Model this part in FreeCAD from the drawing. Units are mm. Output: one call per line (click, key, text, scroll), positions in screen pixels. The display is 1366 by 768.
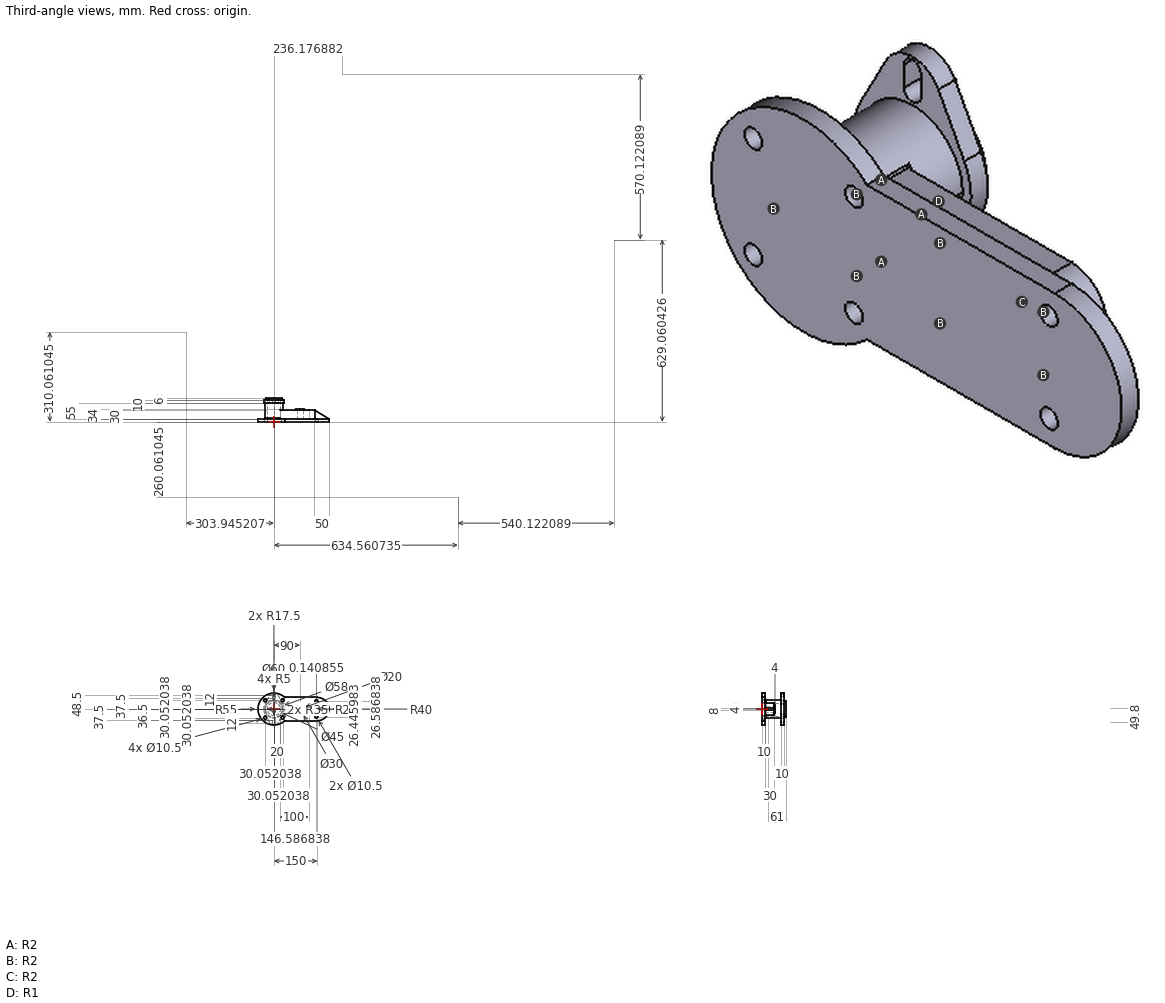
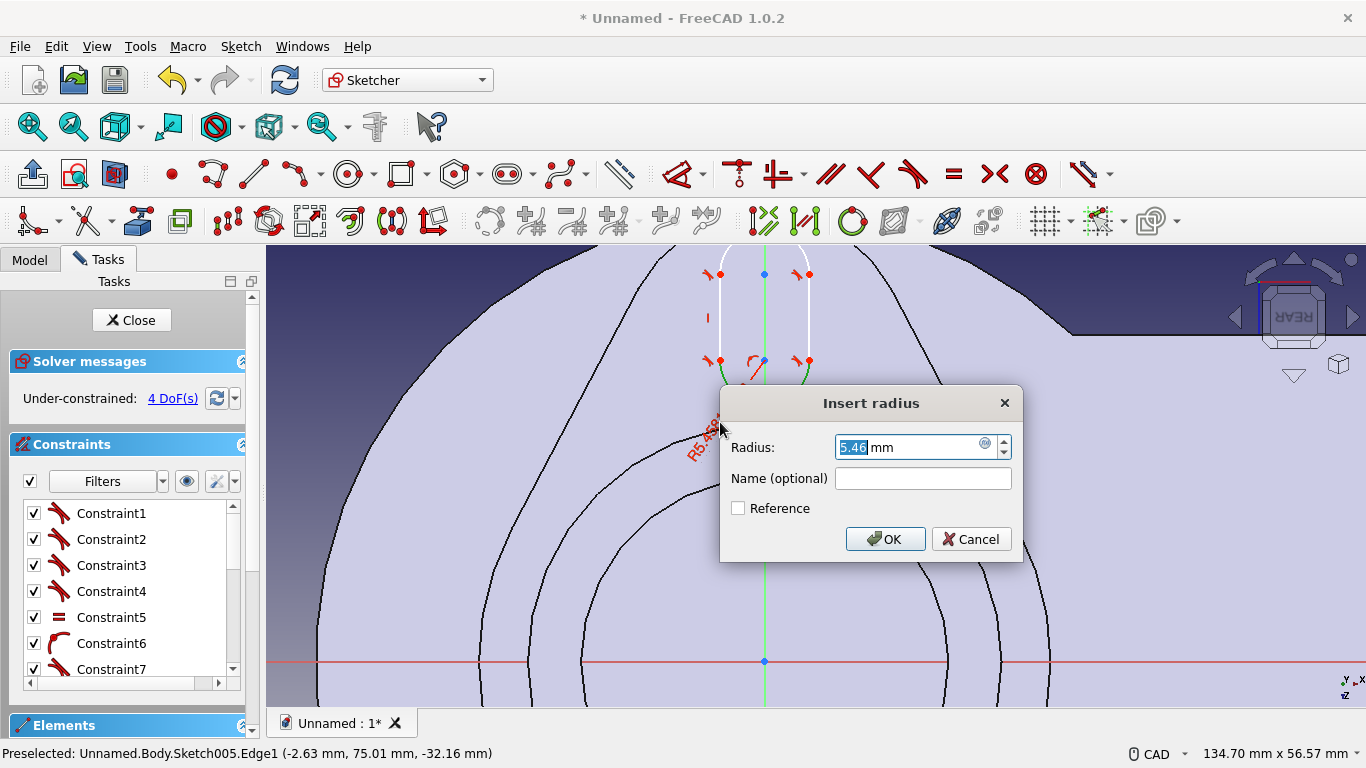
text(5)
key(Return)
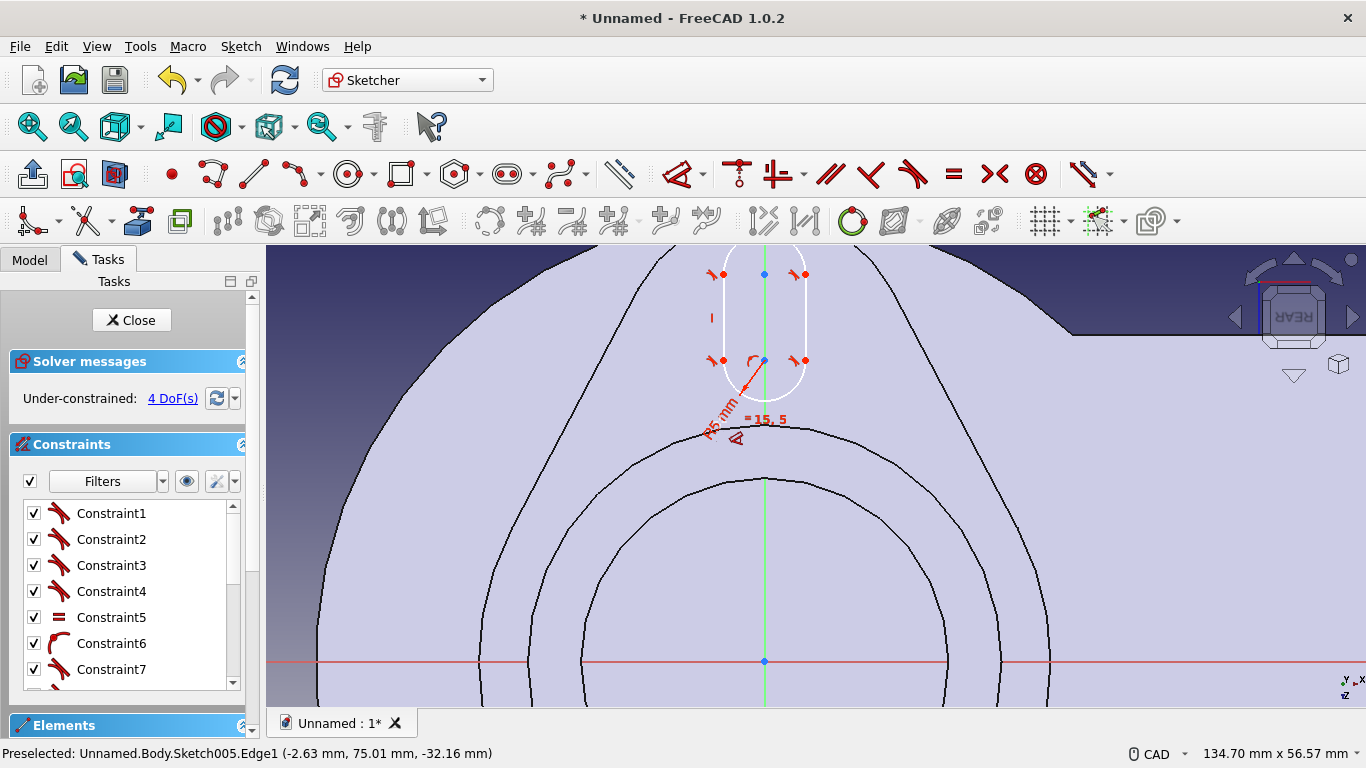
click(724, 334)
click(690, 317)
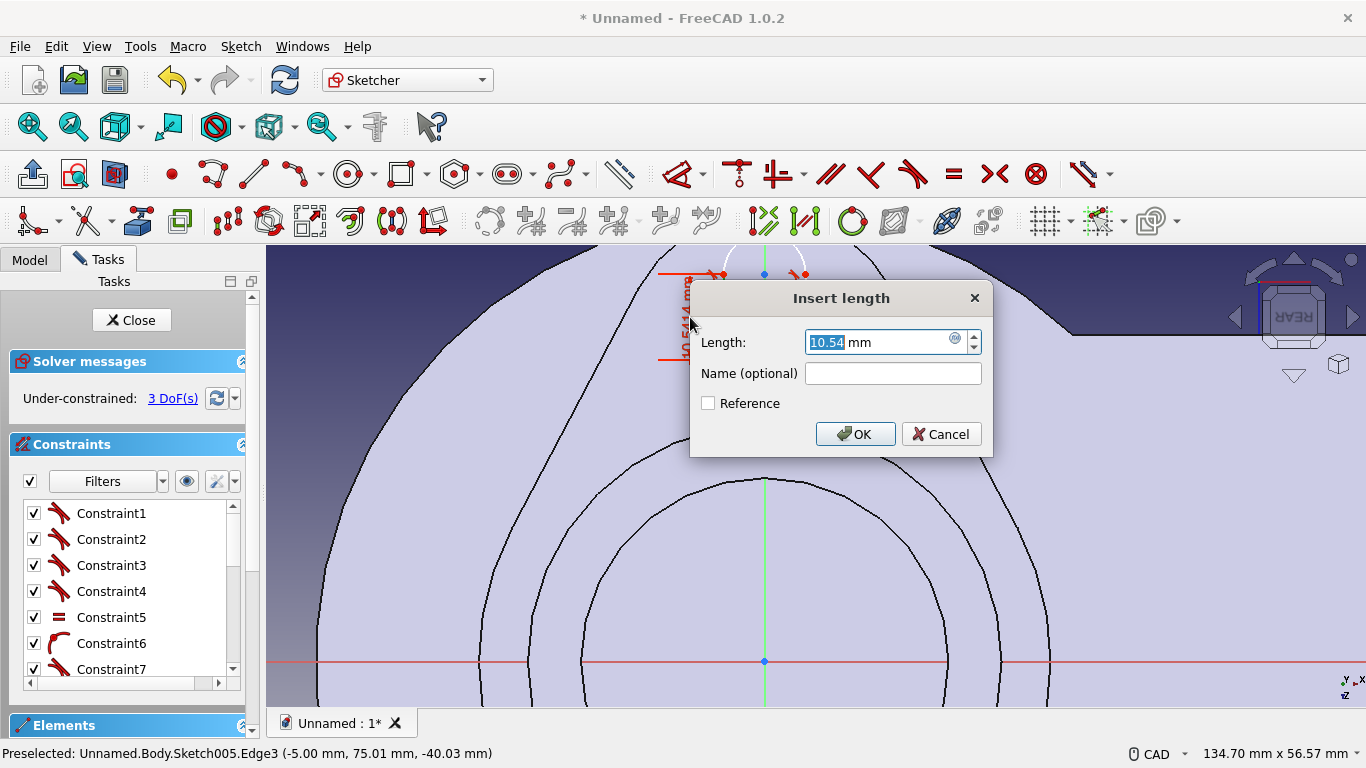
text(12)
key(Return)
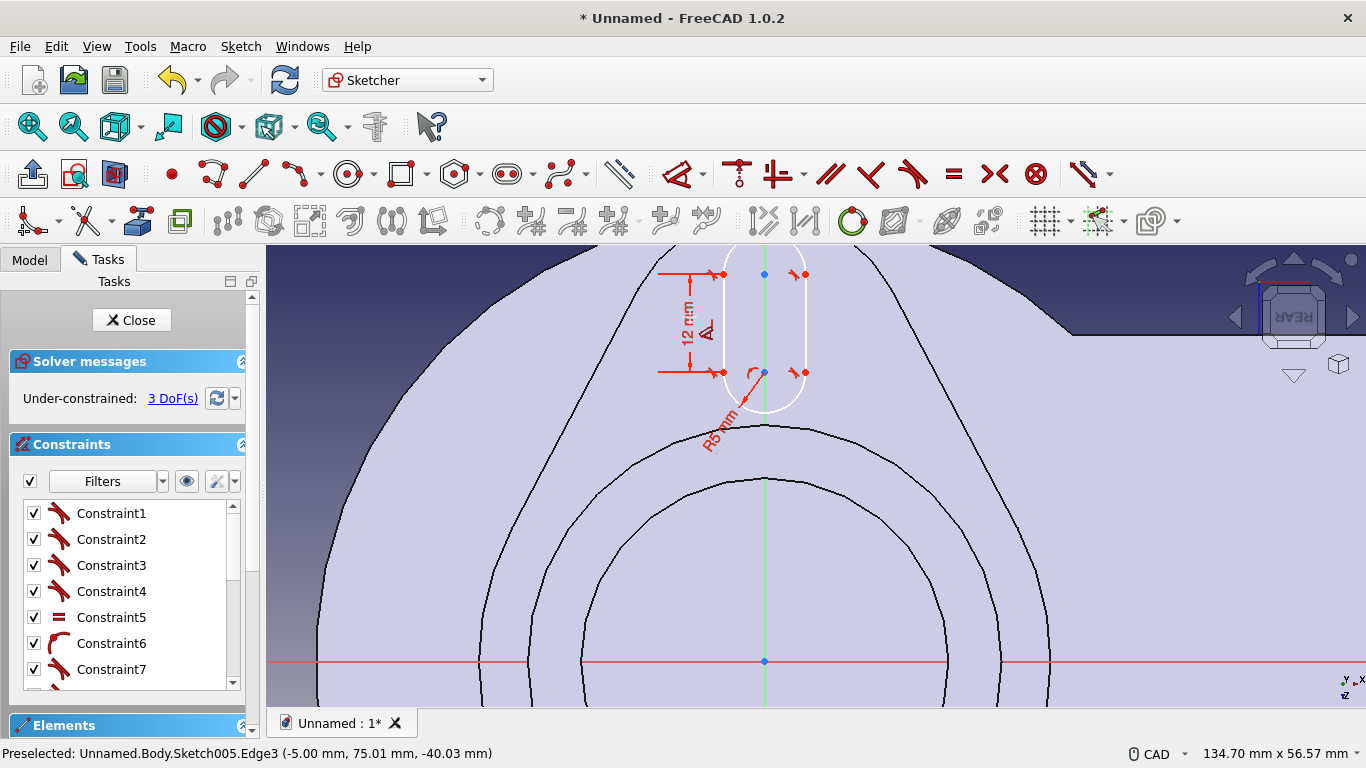
scroll(740, 396, down, 6)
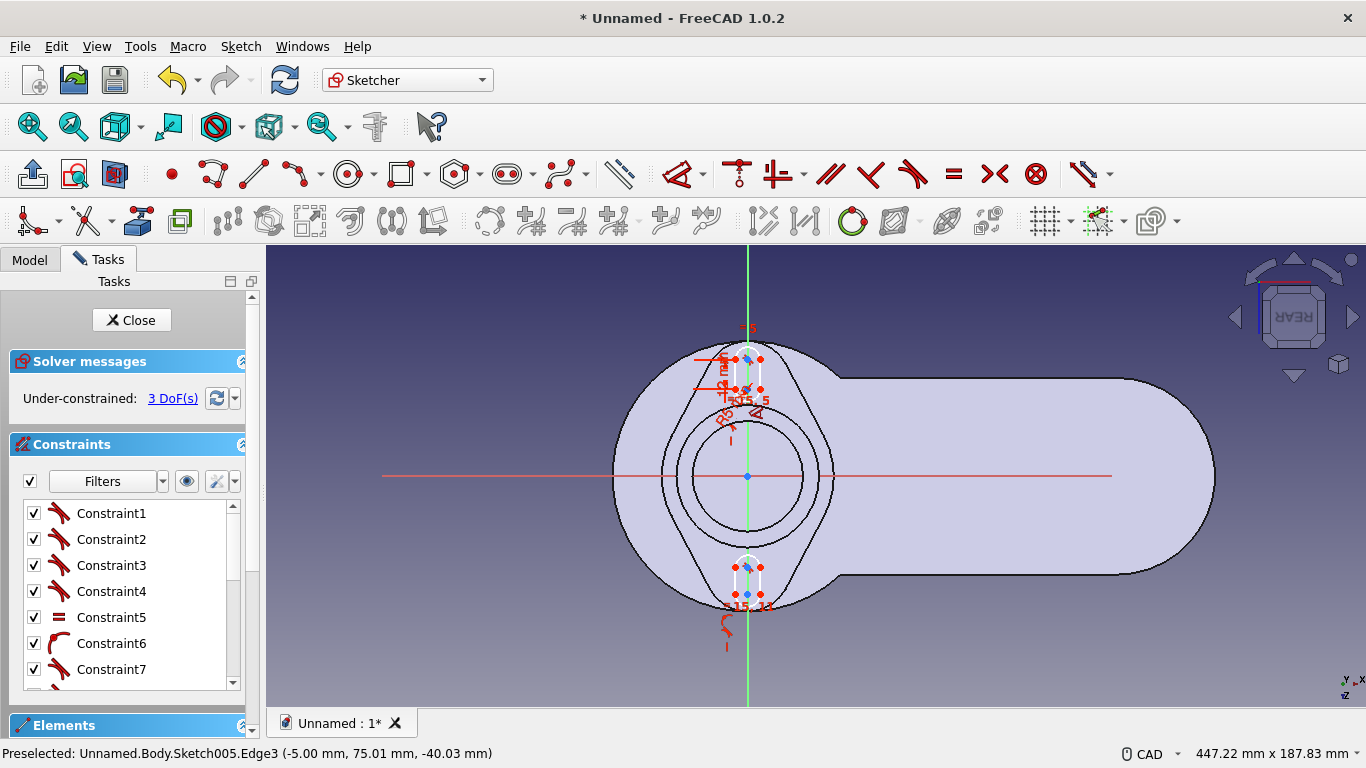
scroll(735, 586, up, 3)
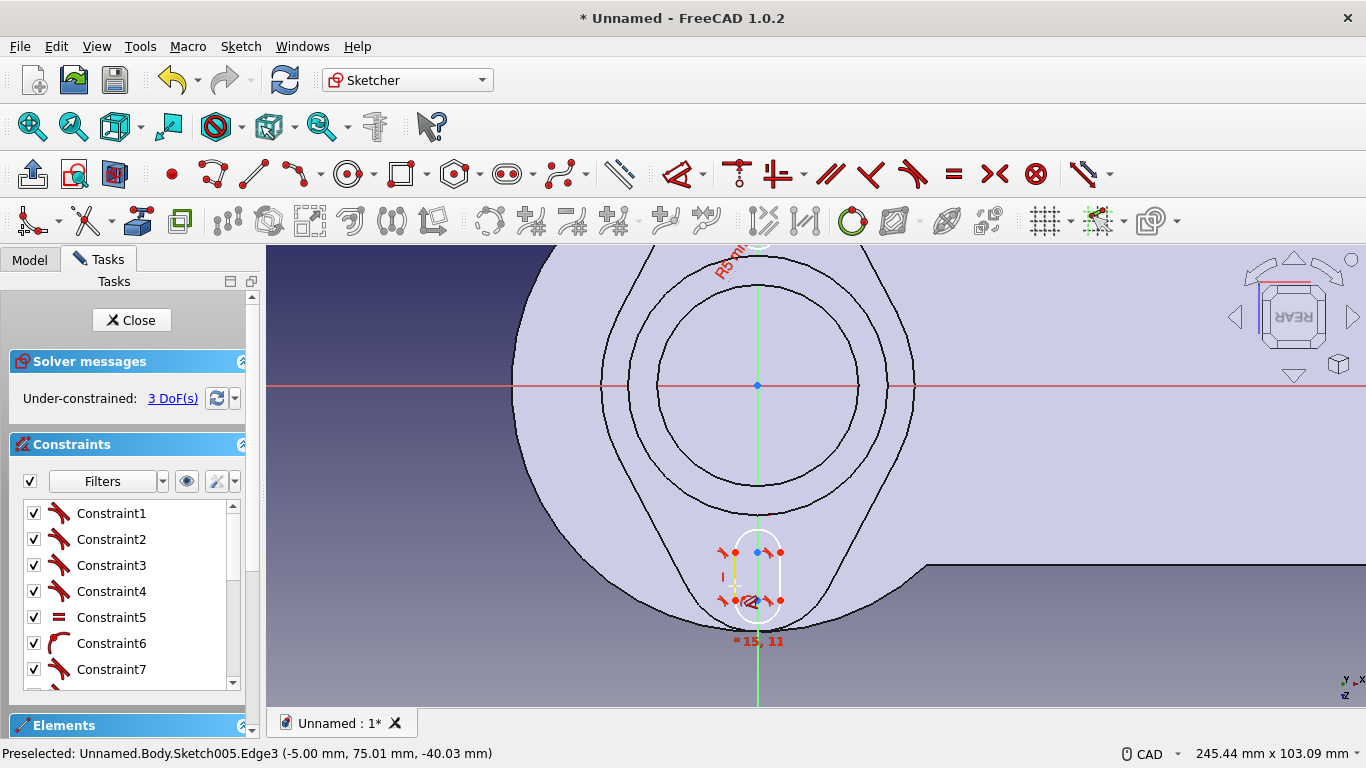
click(735, 586)
click(701, 576)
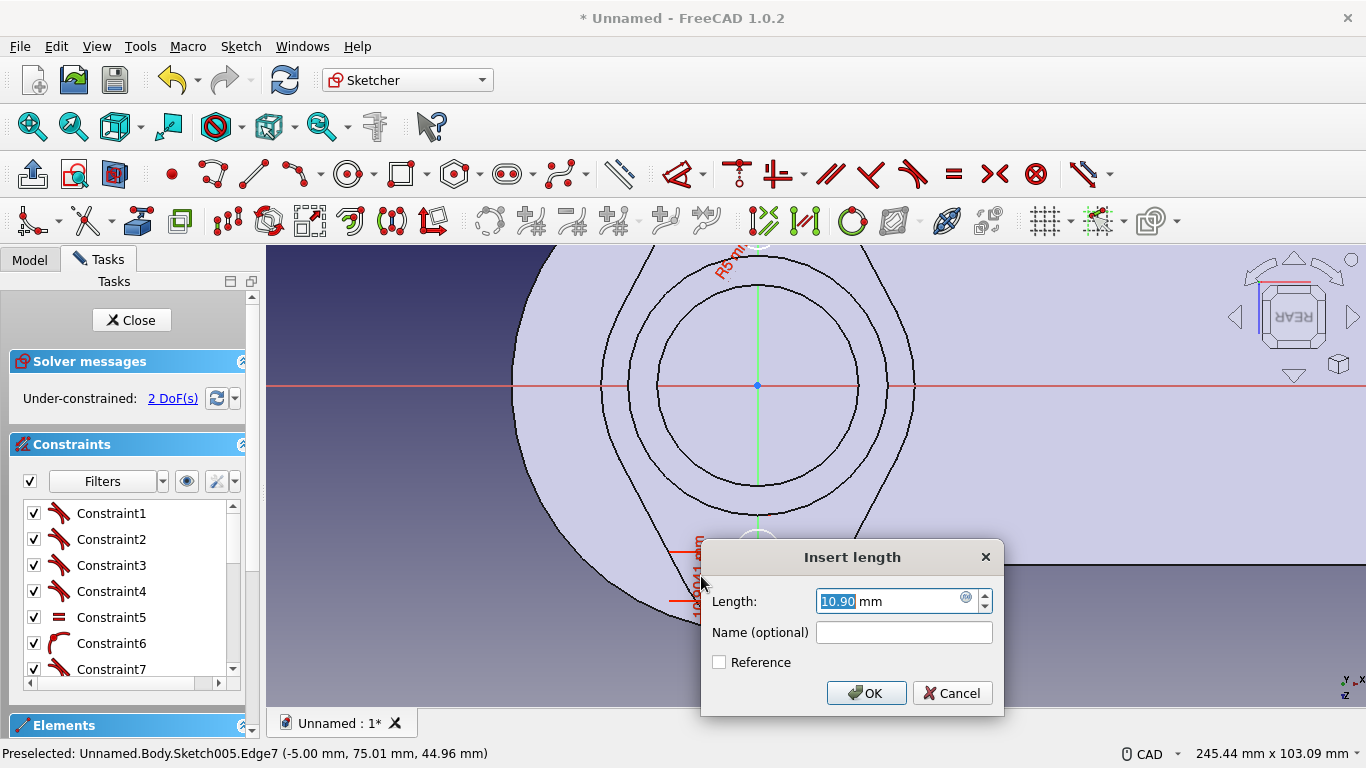
text(12)
key(Return)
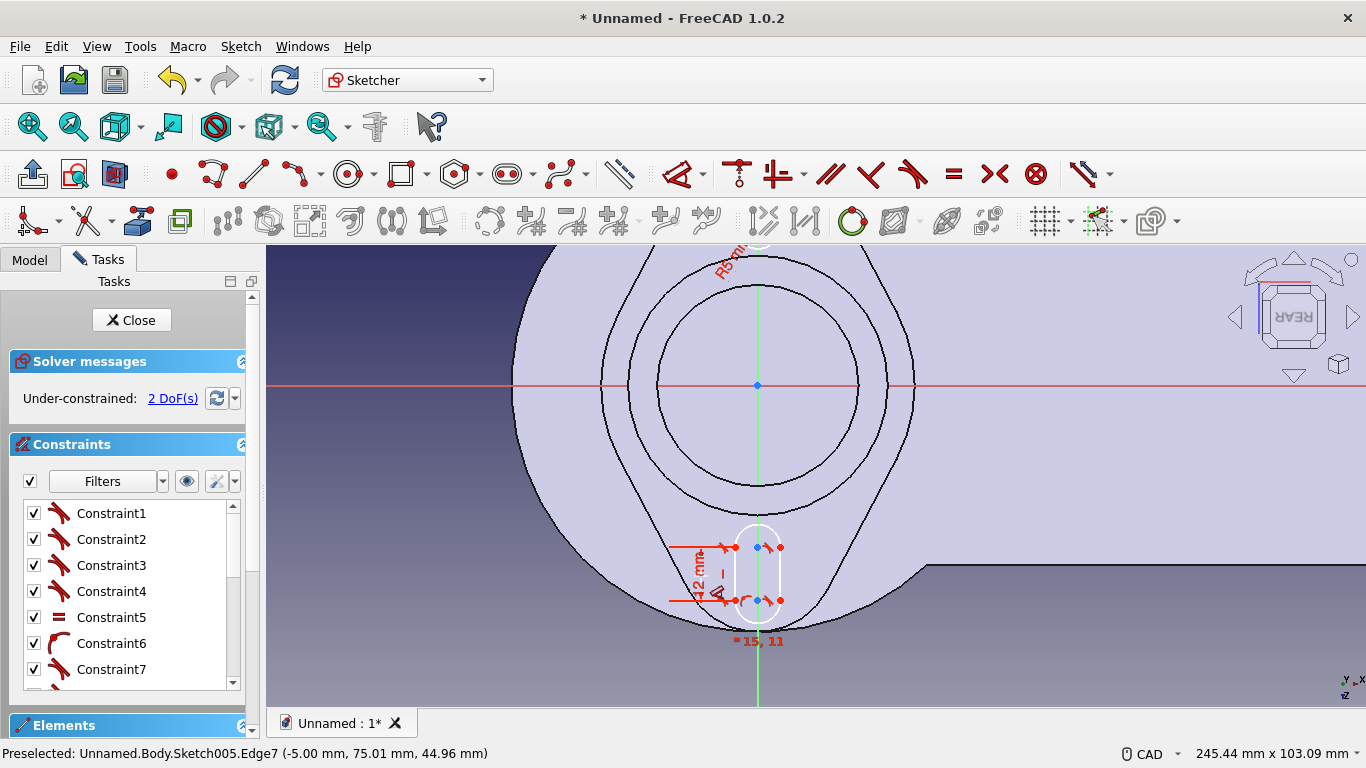
scroll(735, 586, down, 3)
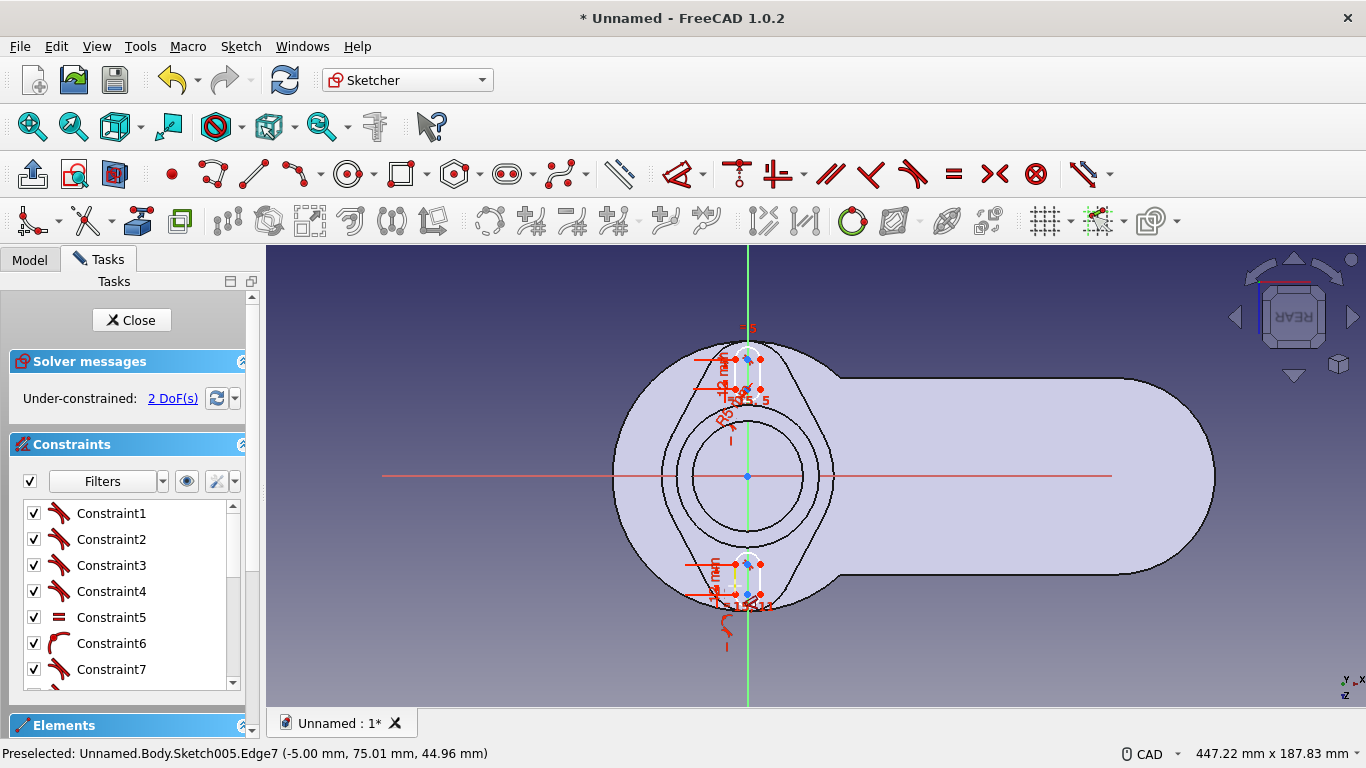
click(735, 389)
click(701, 433)